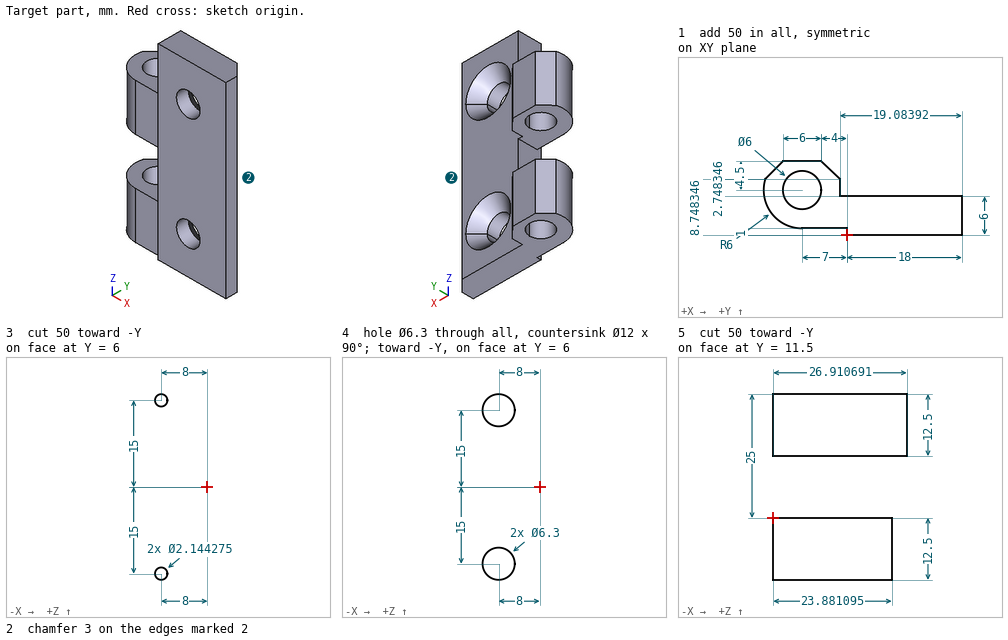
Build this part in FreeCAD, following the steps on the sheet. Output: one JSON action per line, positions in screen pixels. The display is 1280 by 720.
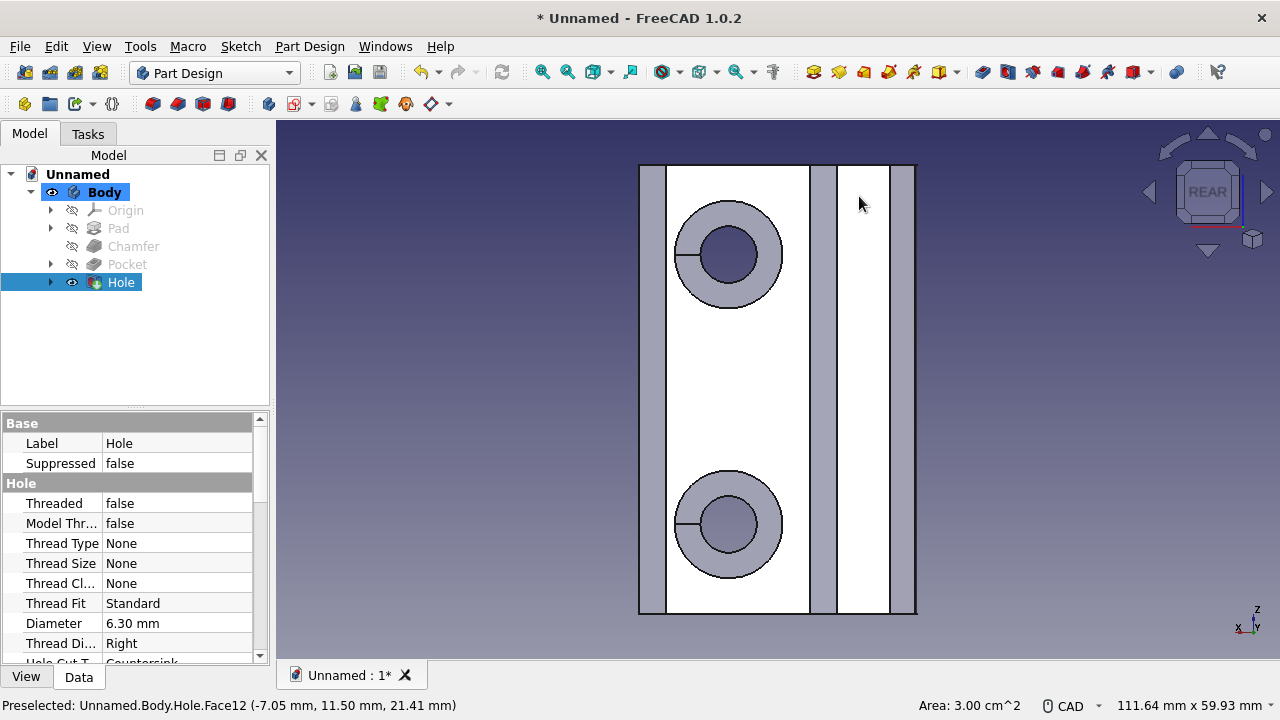
{"action": "left_click", "coordinate": [294, 104]}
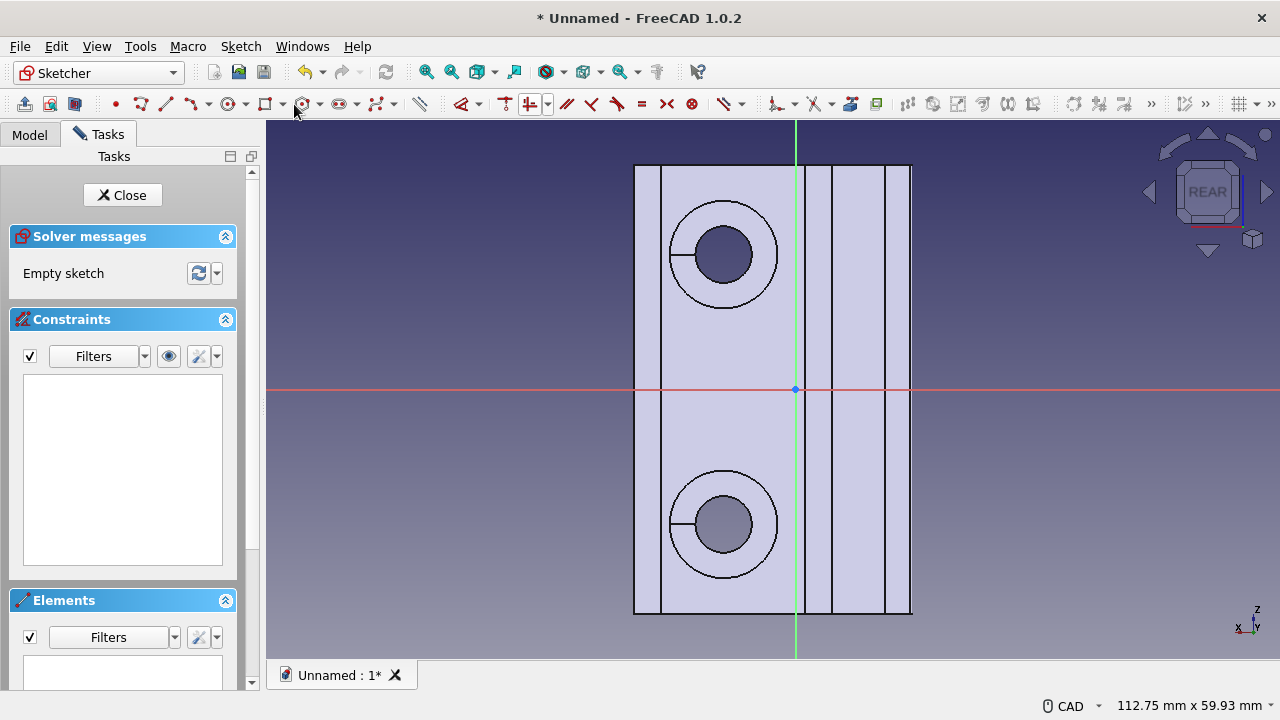
{"action": "scroll", "coordinate": [294, 631], "scroll_direction": "down", "scroll_amount": 1}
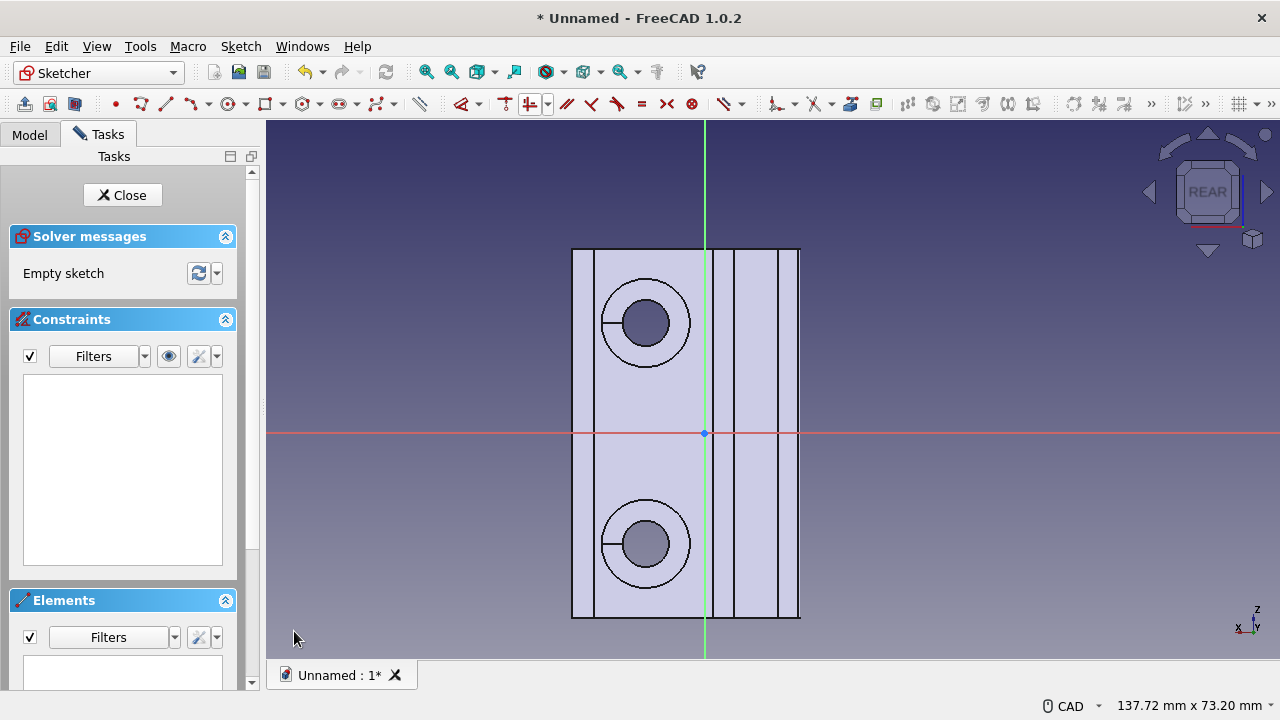
{"action": "left_click", "coordinate": [264, 104]}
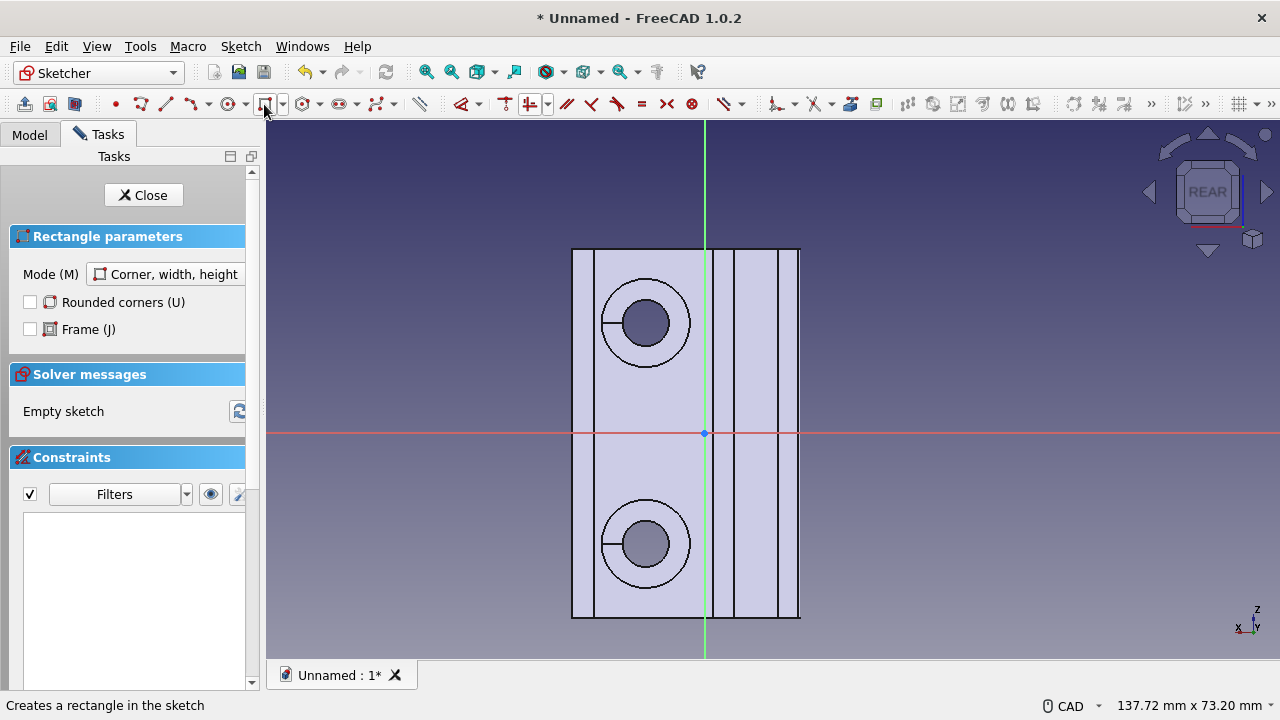
{"action": "left_click", "coordinate": [705, 433]}
{"action": "mouse_move", "coordinate": [880, 525]}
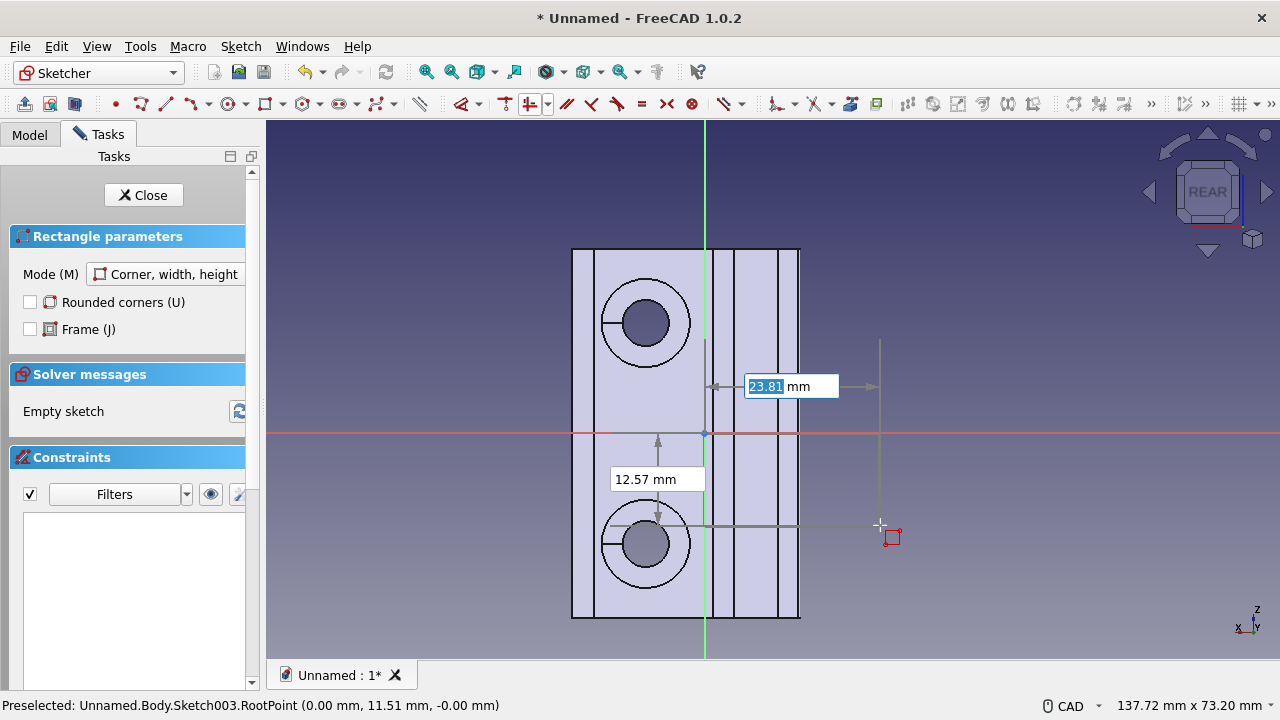
{"action": "type", "text": "23.881095"}
{"action": "key", "text": "Tab"}
{"action": "type", "text": "12.5"}
{"action": "key", "text": "Return"}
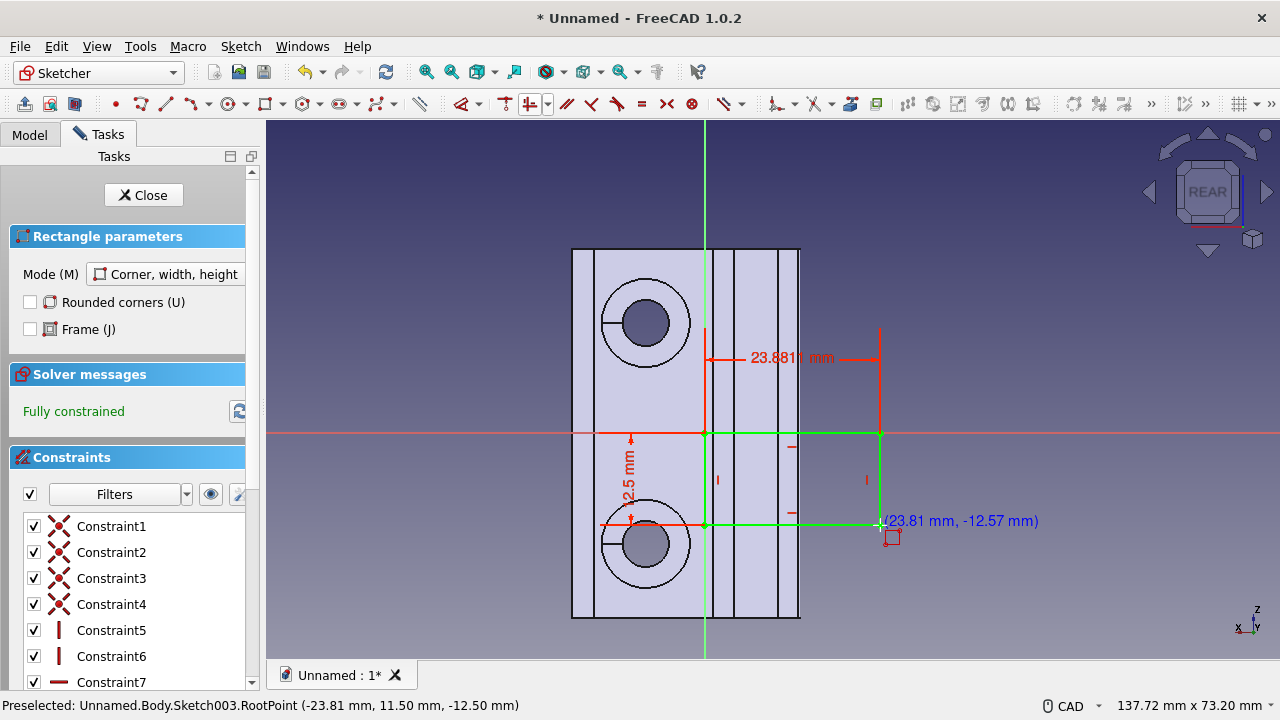
{"action": "left_click", "coordinate": [705, 249]}
{"action": "mouse_move", "coordinate": [903, 341]}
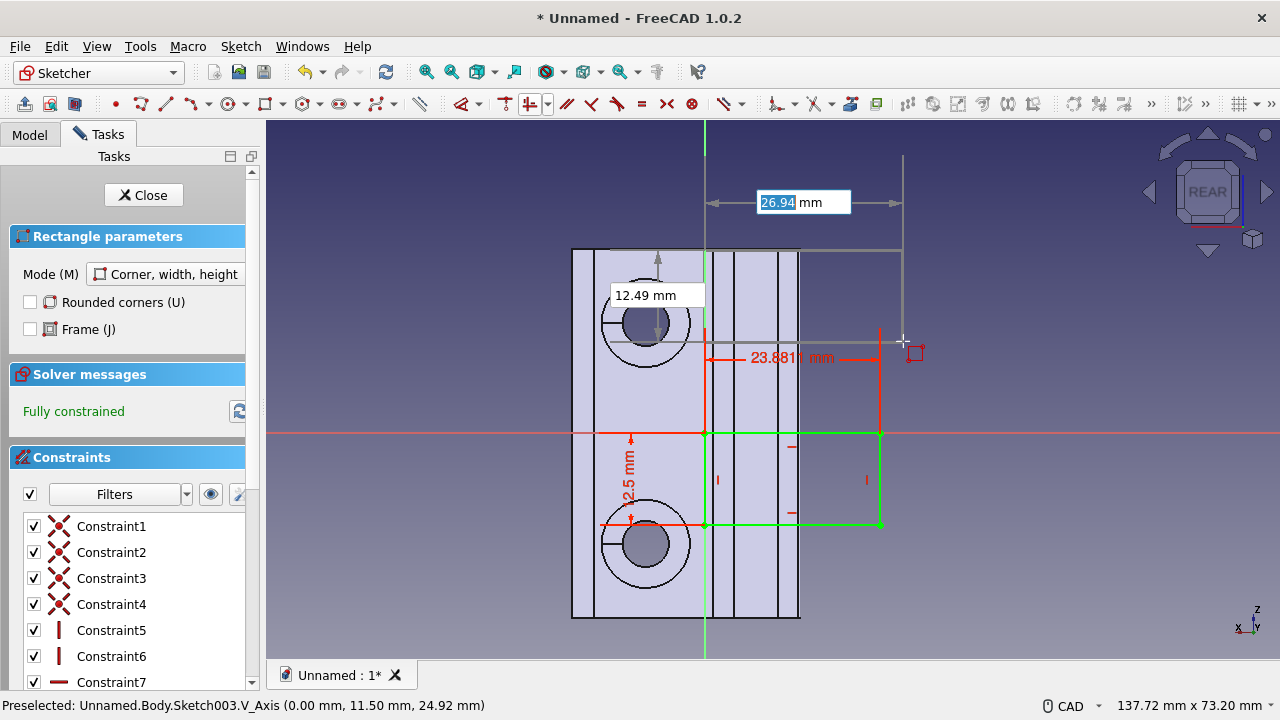
{"action": "type", "text": "26.910691"}
{"action": "key", "text": "Tab"}
{"action": "type", "text": "12.5"}
{"action": "key", "text": "Return"}
{"action": "key", "text": "Escape"}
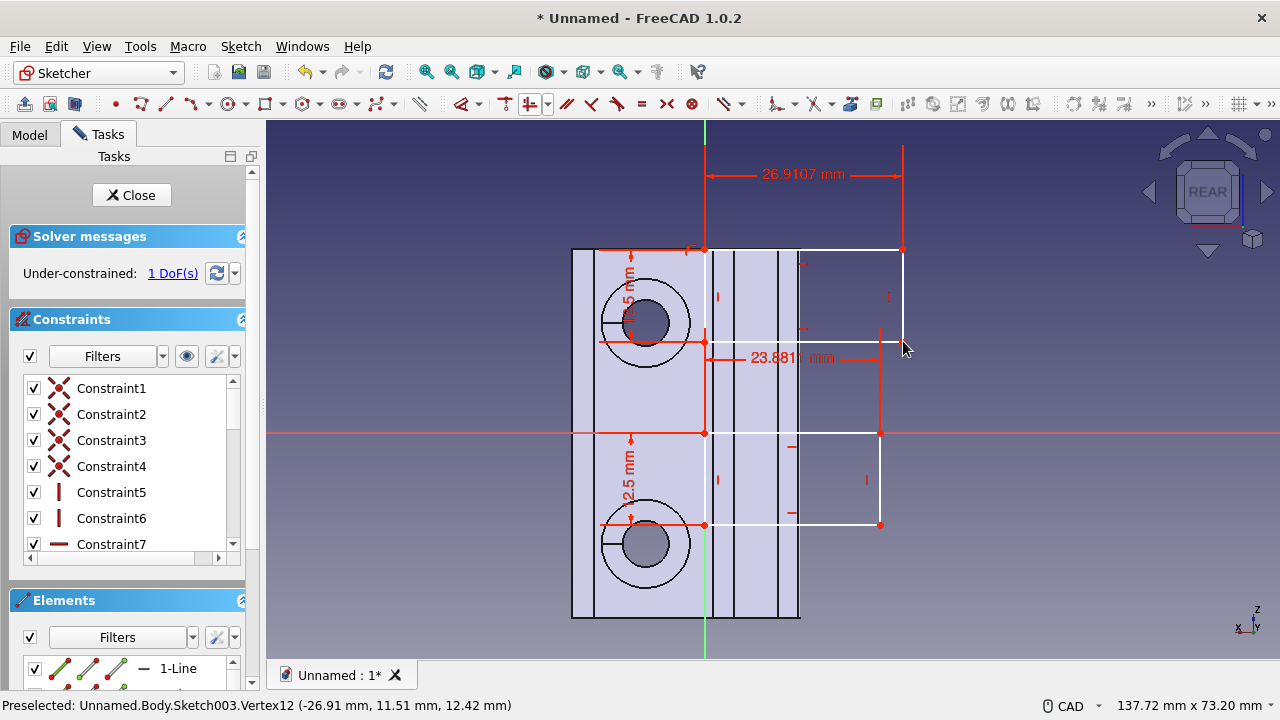
{"action": "key", "text": "d"}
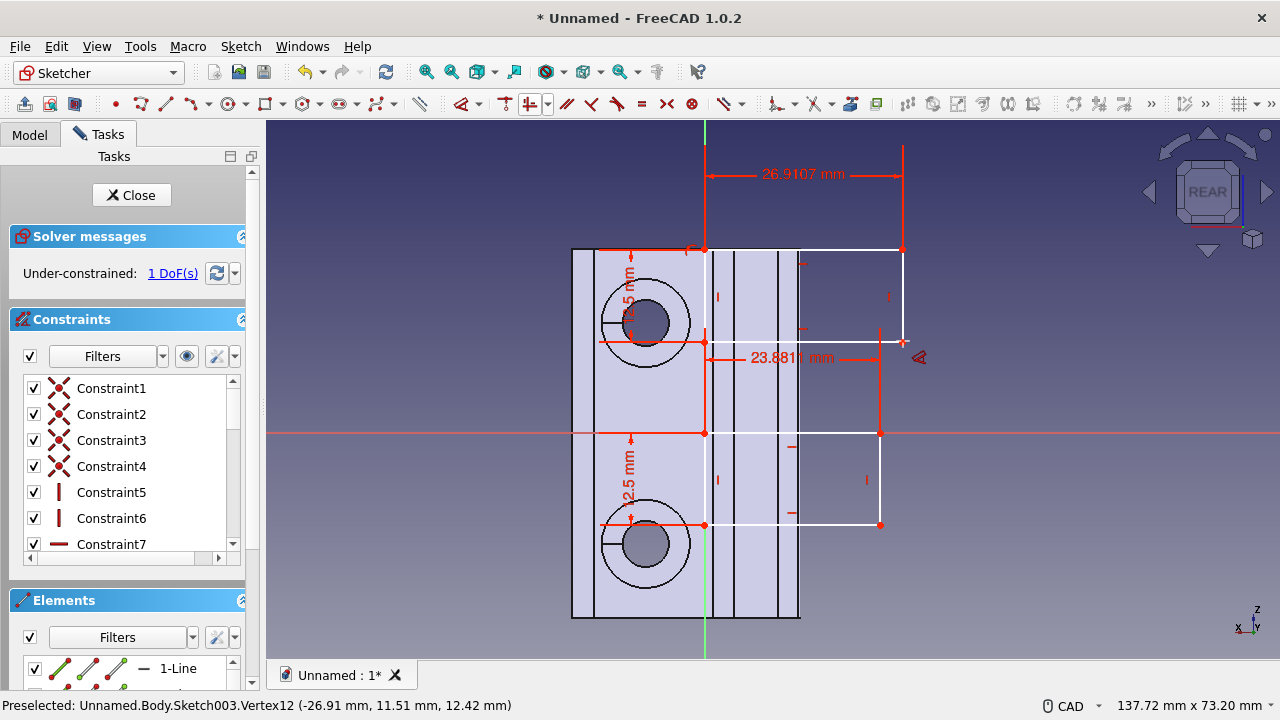
{"action": "left_click", "coordinate": [705, 250]}
{"action": "left_click", "coordinate": [671, 342]}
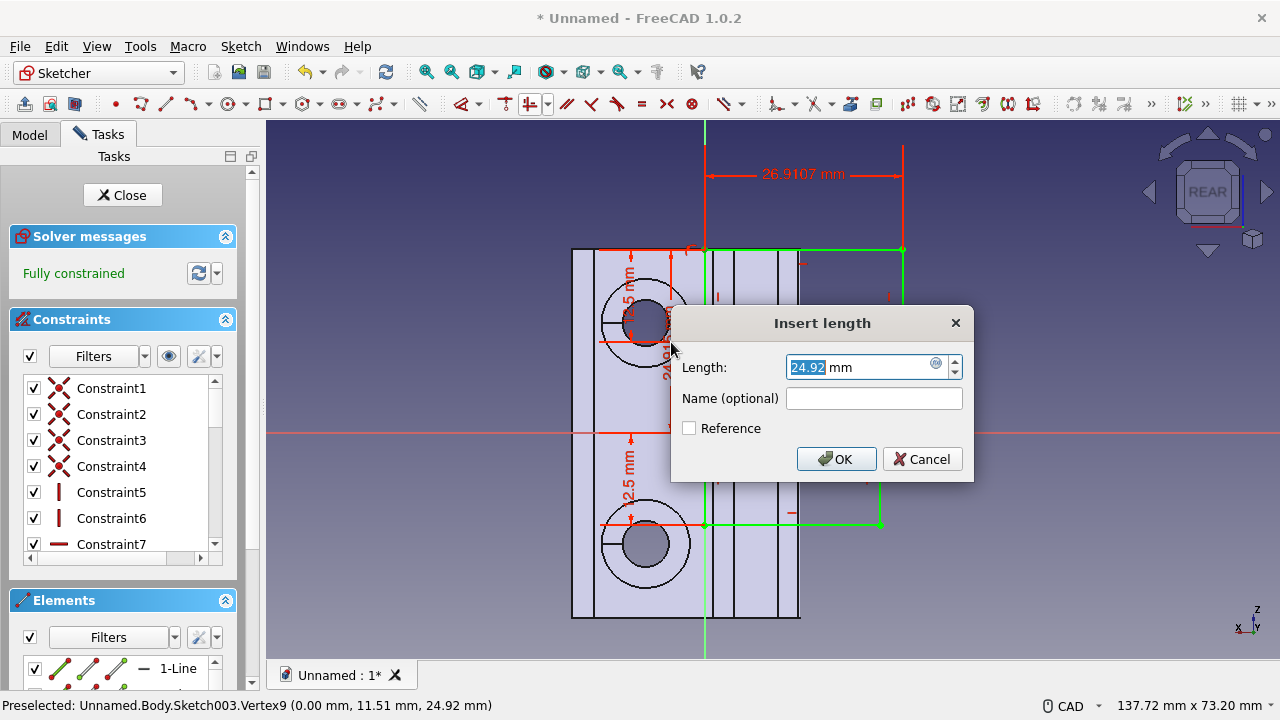
{"action": "type", "text": "25"}
{"action": "key", "text": "Return"}
{"action": "key", "text": "Escape"}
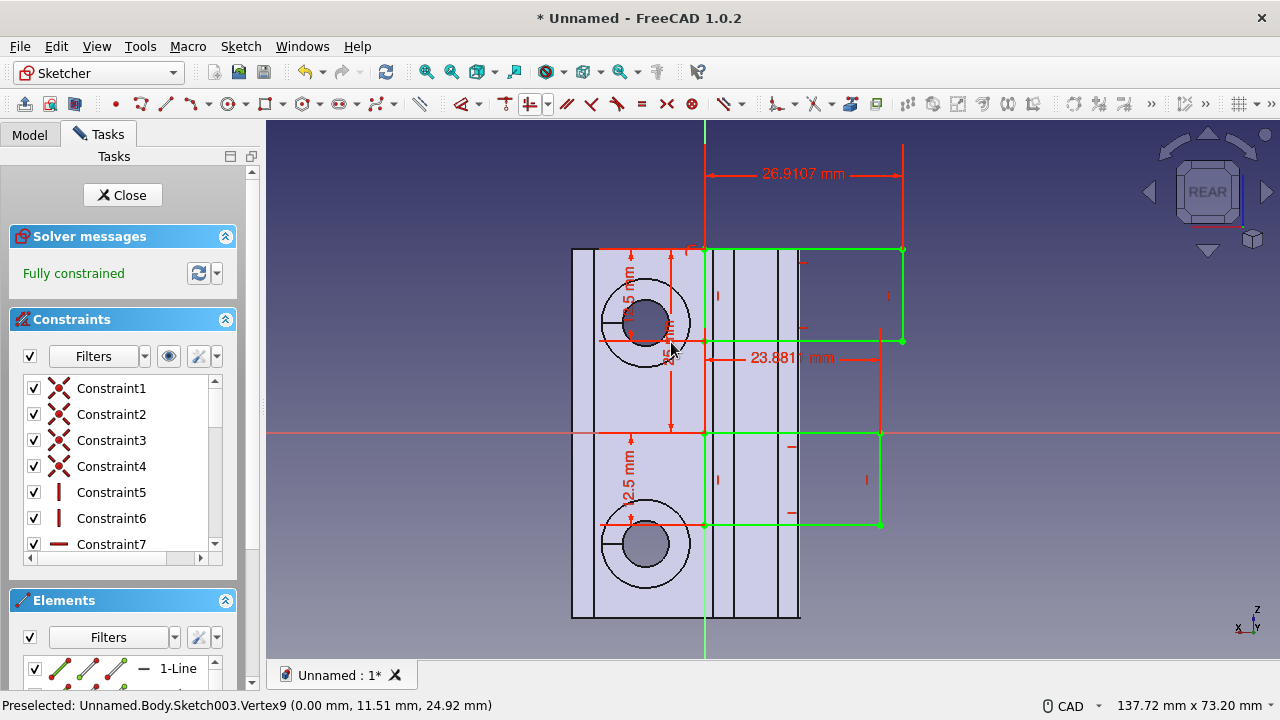
{"action": "left_click", "coordinate": [123, 195]}